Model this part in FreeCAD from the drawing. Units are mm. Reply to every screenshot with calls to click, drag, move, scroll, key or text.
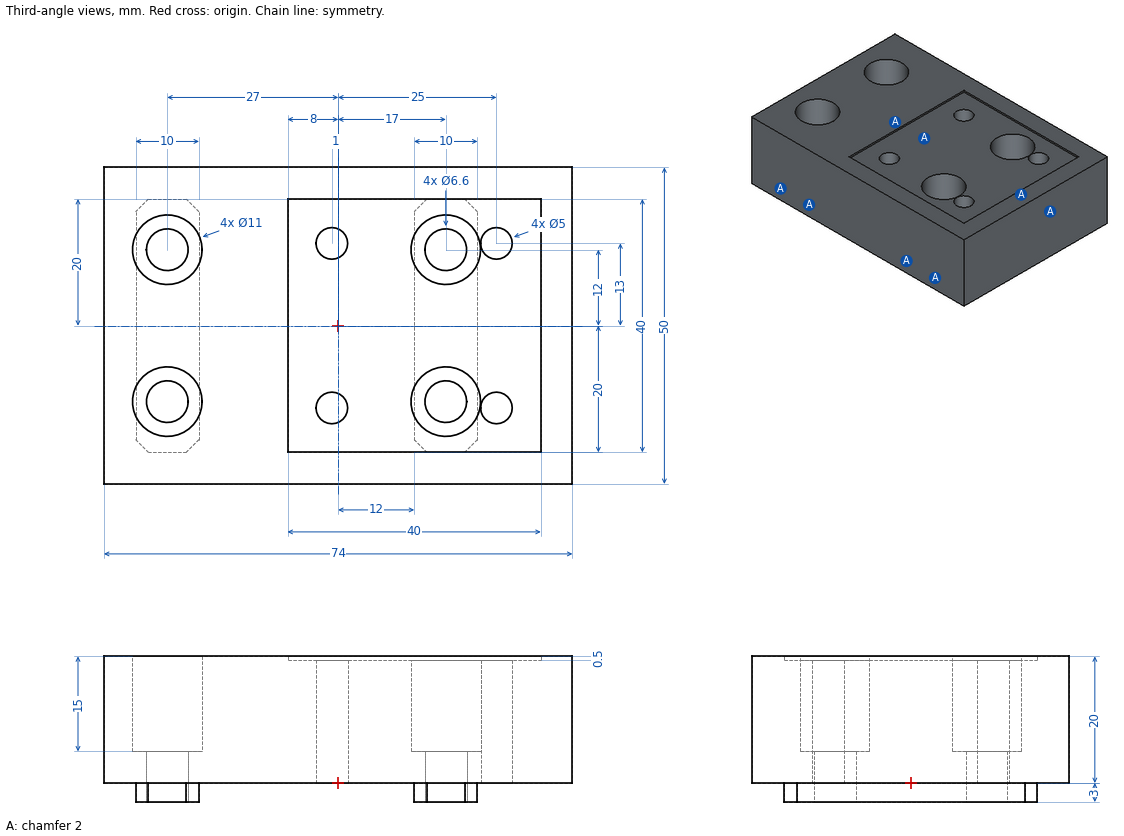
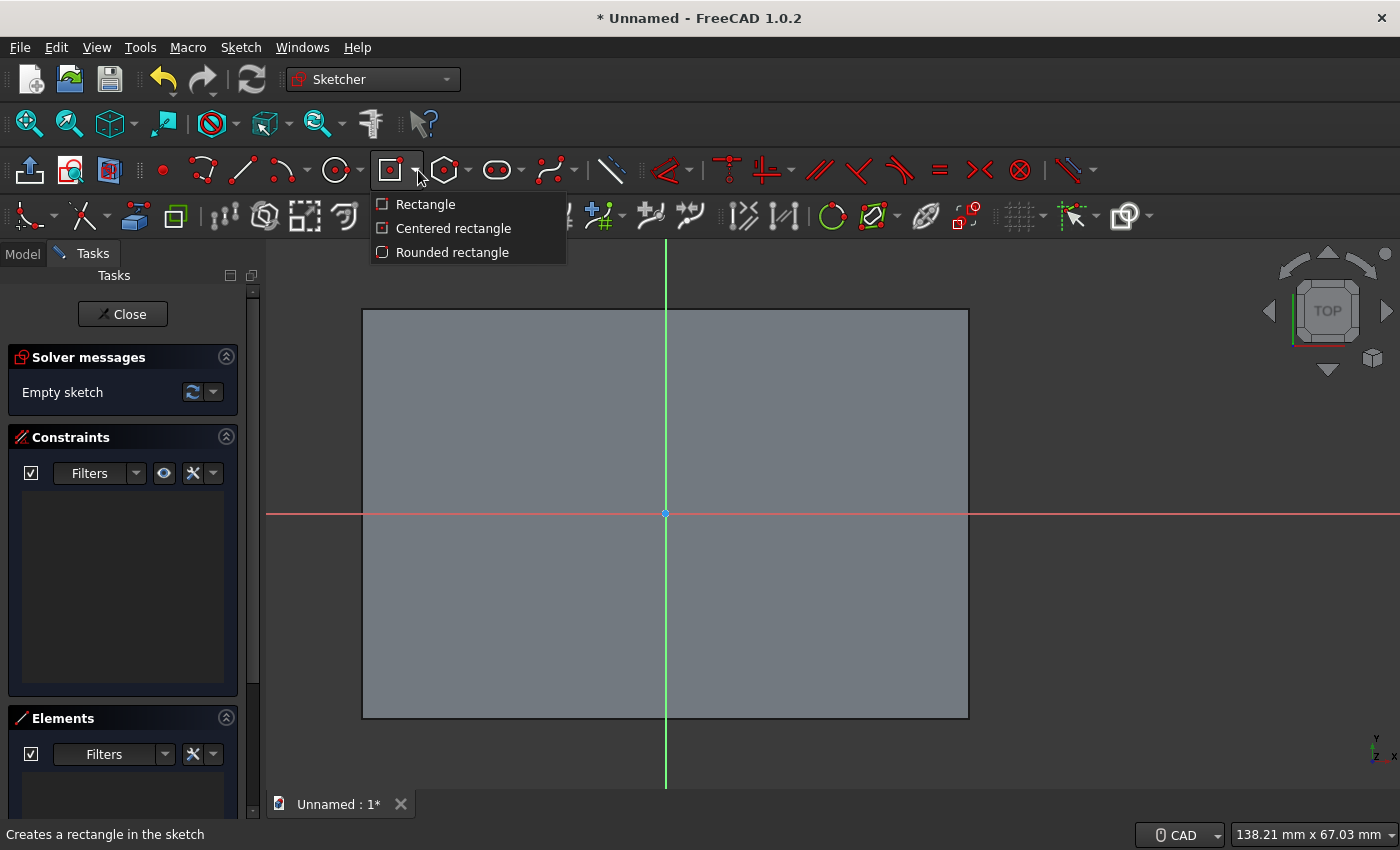
click(468, 204)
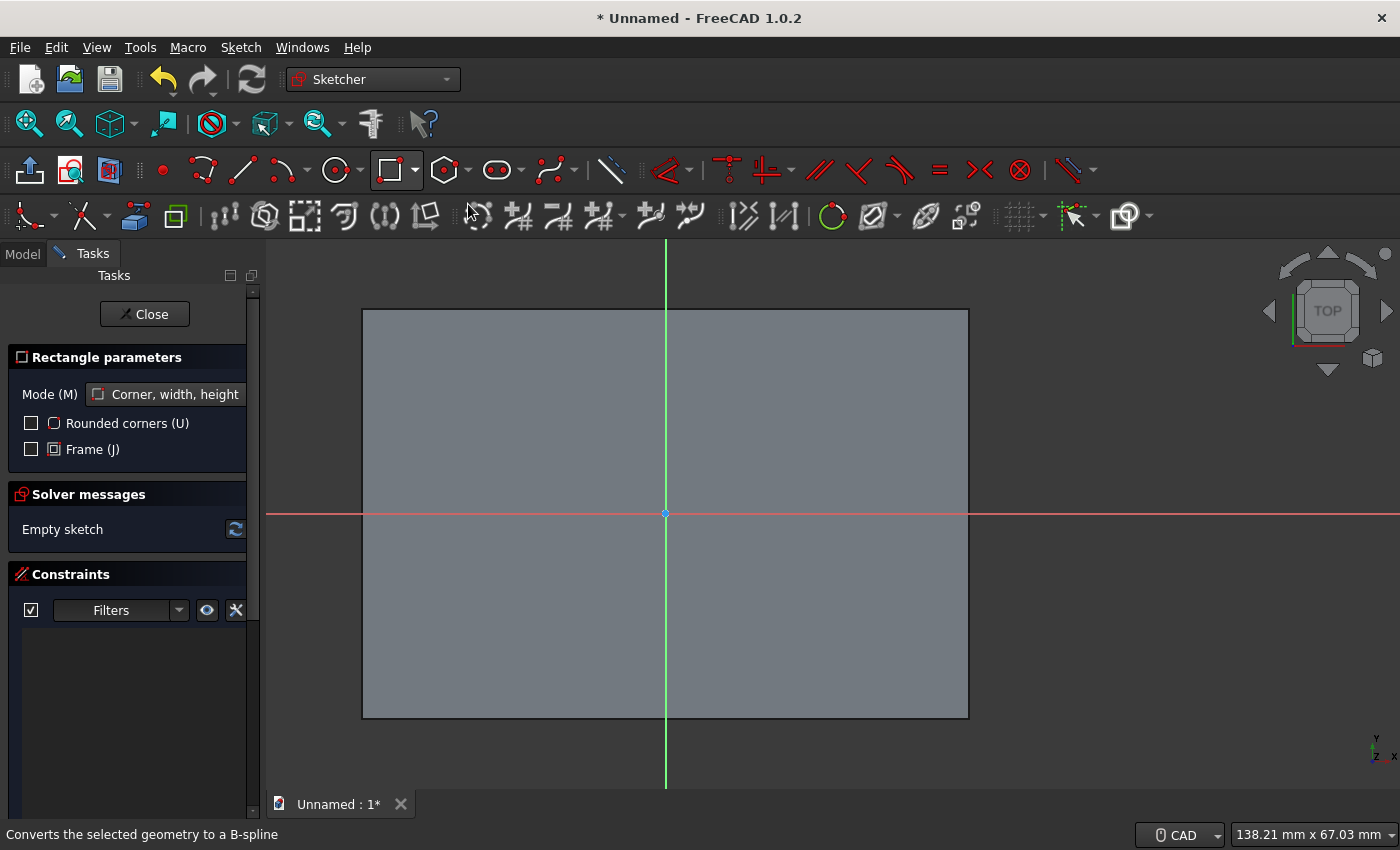
click(600, 350)
move(928, 678)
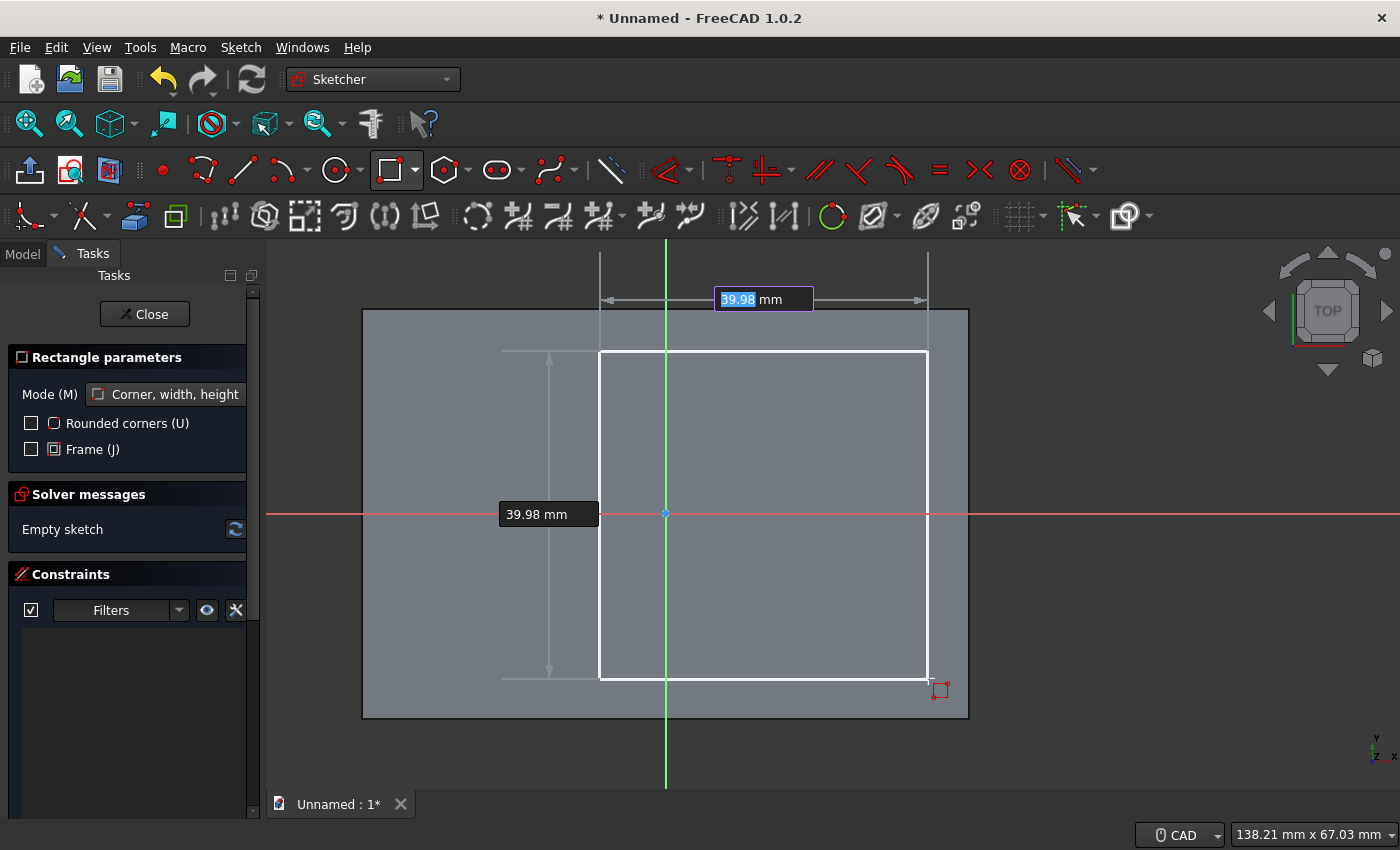
text(40)
key(Tab)
text(40)
key(Return)
key(Escape)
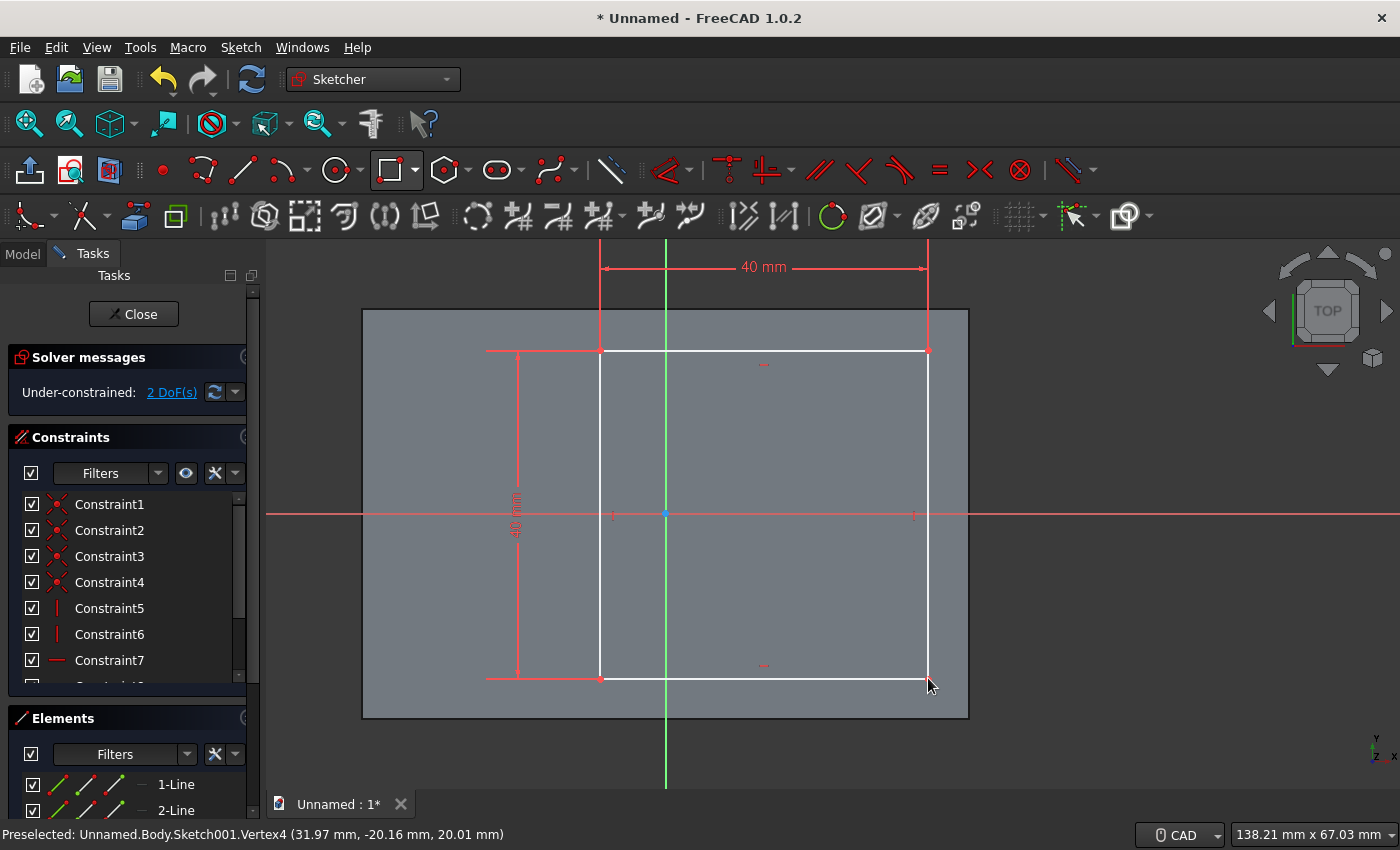
click(666, 170)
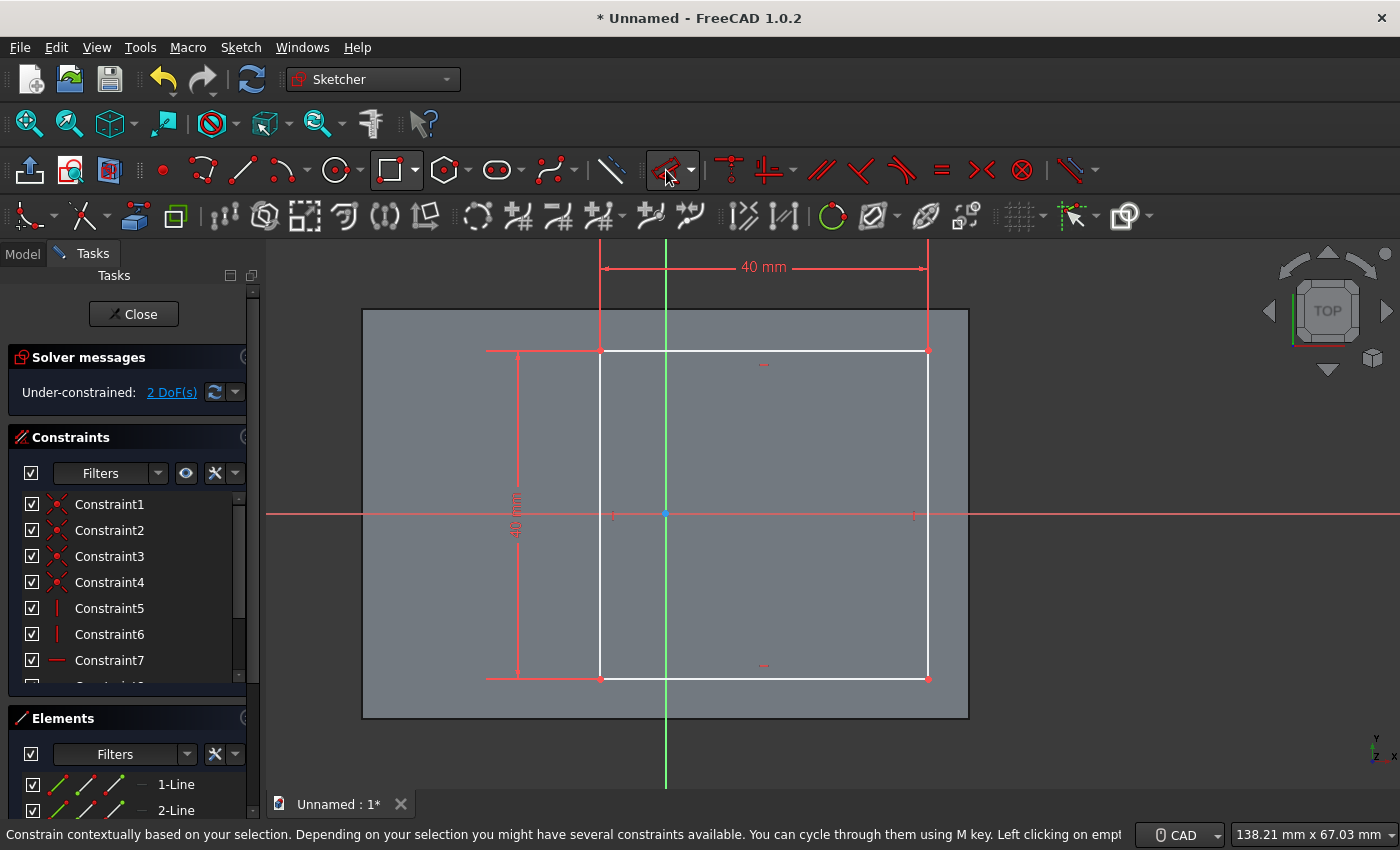
click(600, 351)
click(633, 317)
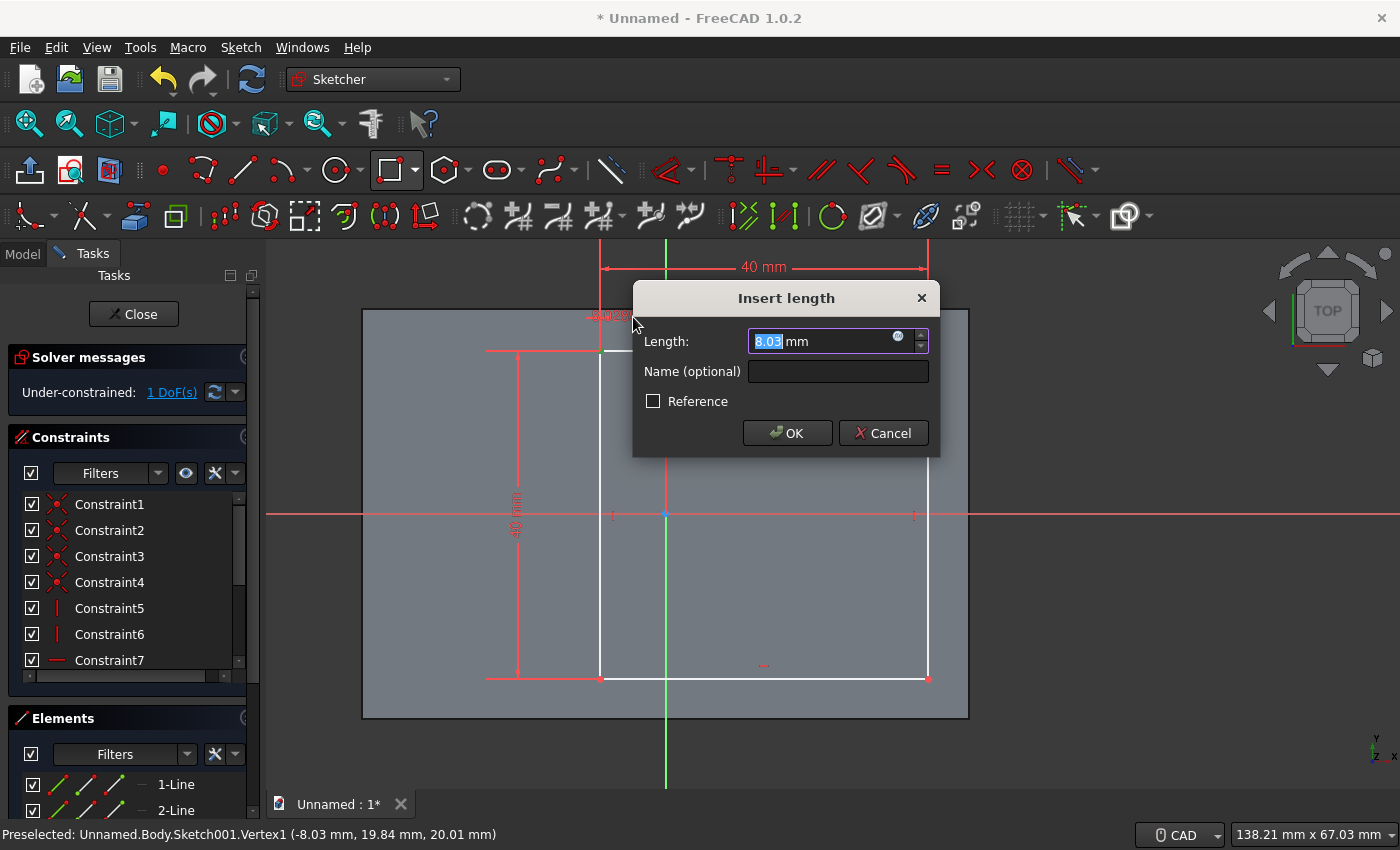
text(8)
key(Return)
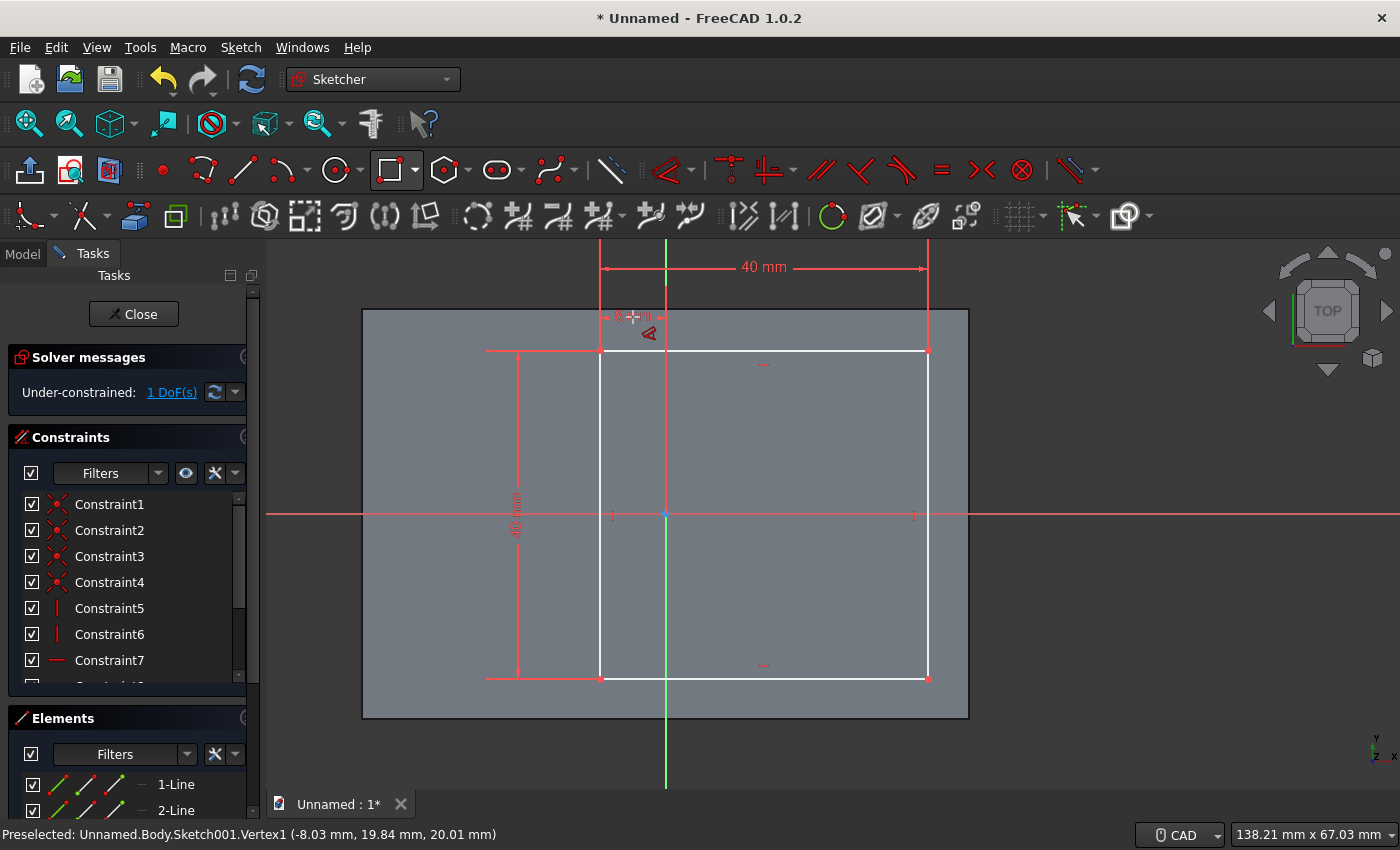
click(600, 351)
click(566, 432)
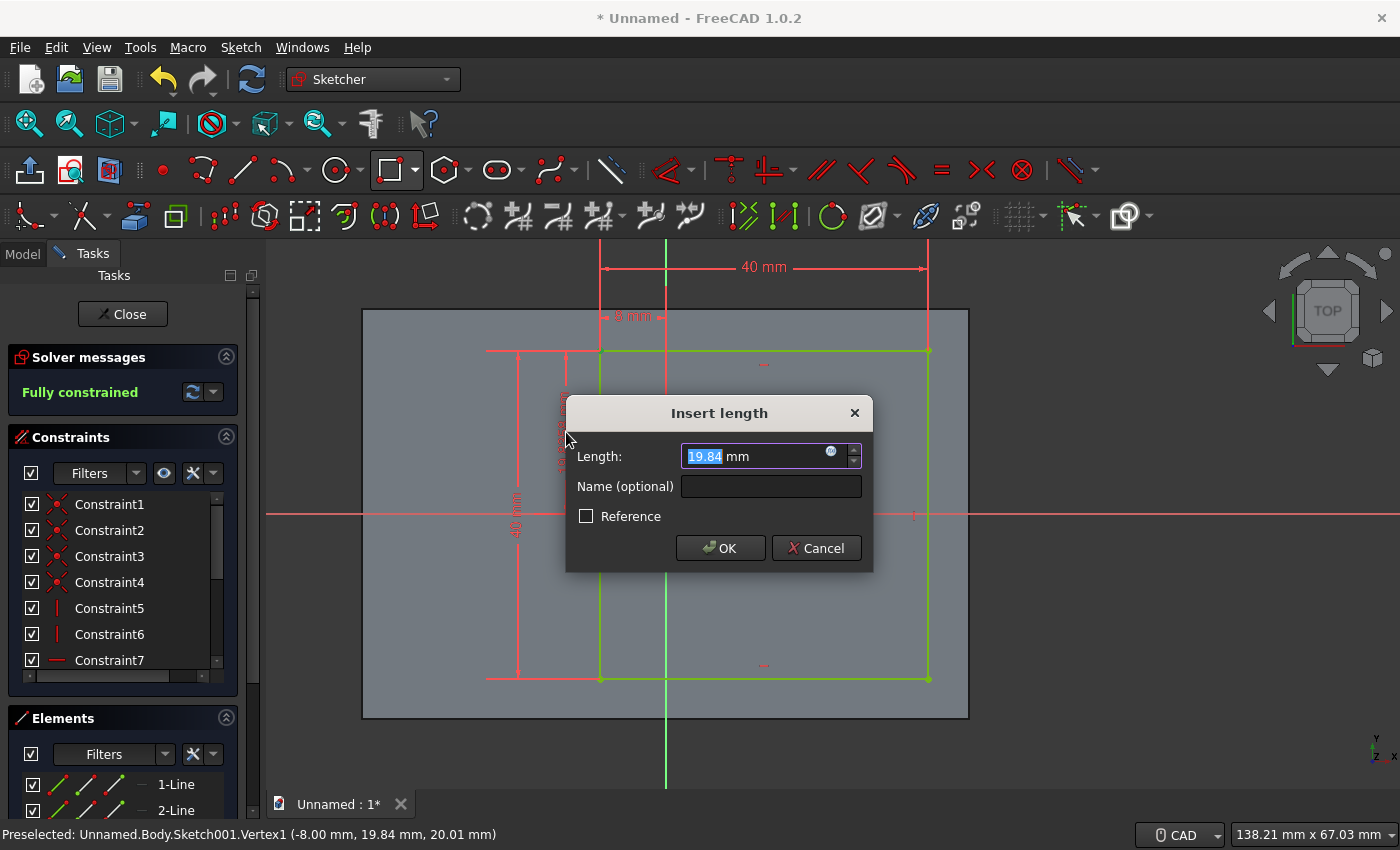
text(20)
key(Return)
key(Escape)